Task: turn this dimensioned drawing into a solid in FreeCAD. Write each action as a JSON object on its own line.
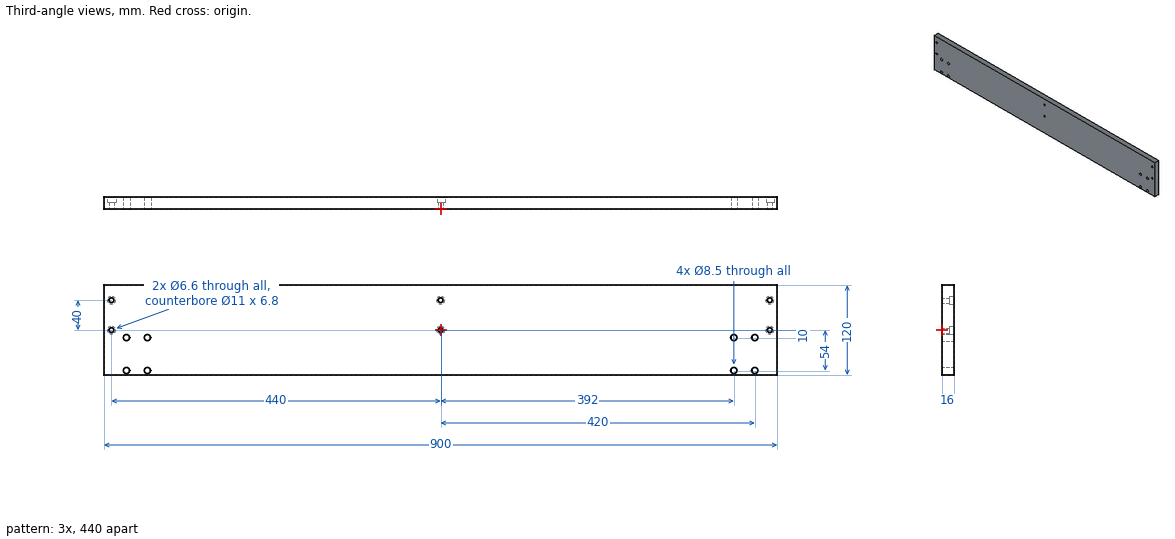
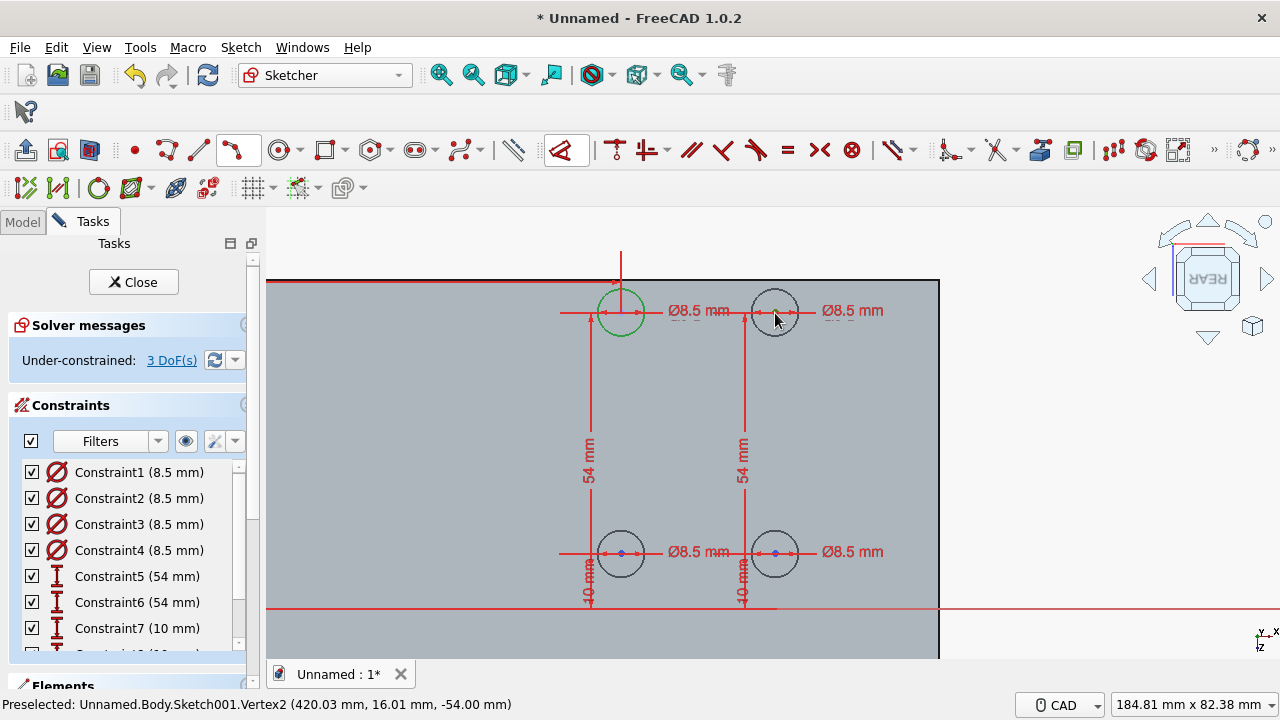
{"action": "key", "text": "l"}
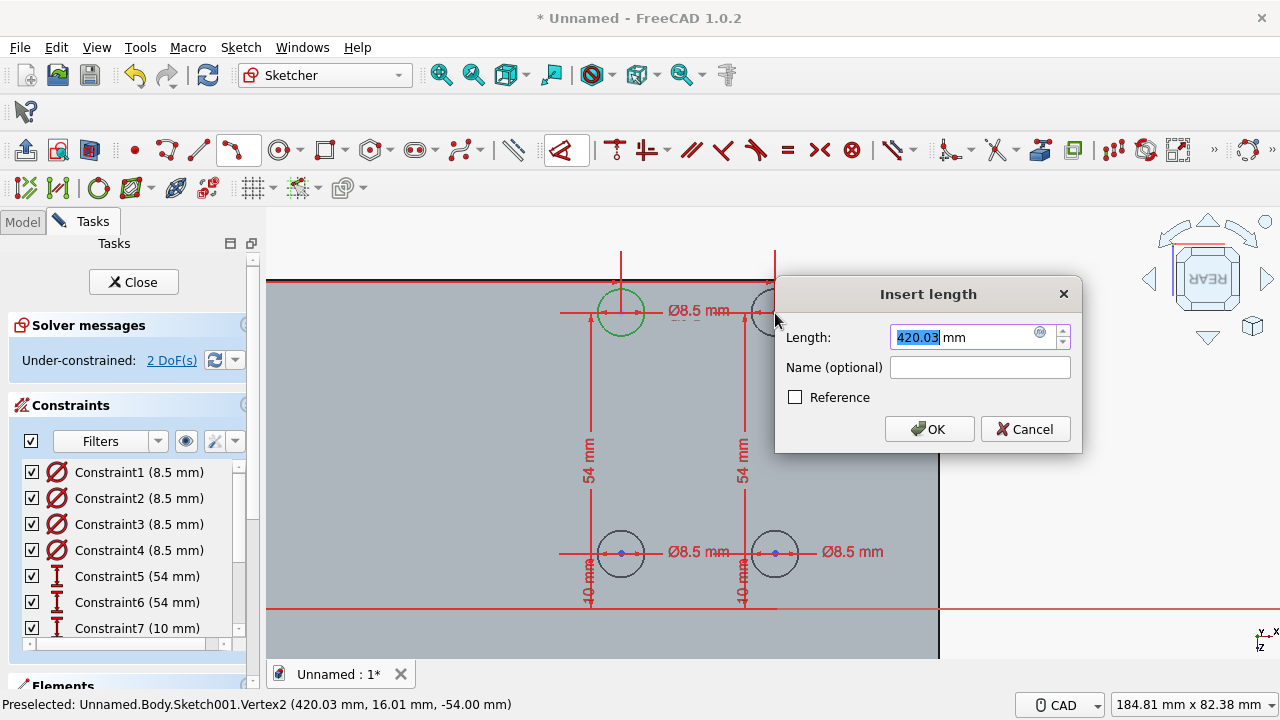
{"action": "type", "text": "420"}
{"action": "key", "text": "Return"}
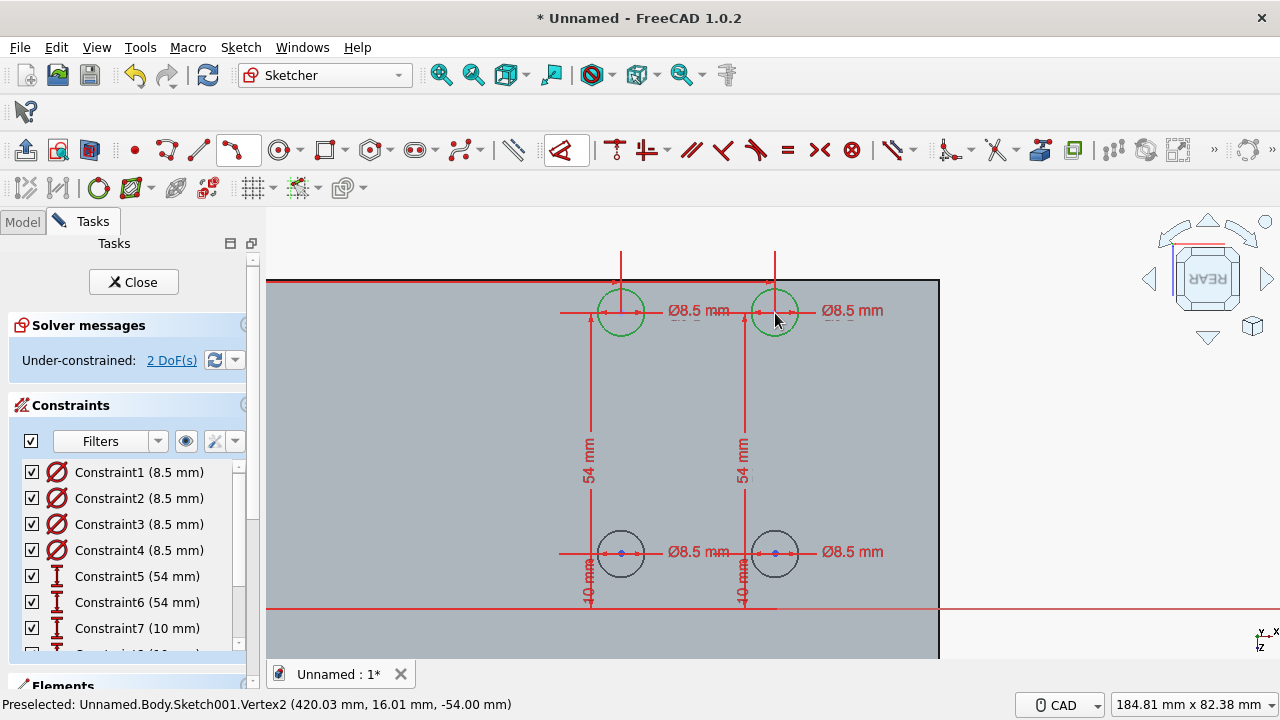
{"action": "left_click", "coordinate": [621, 554]}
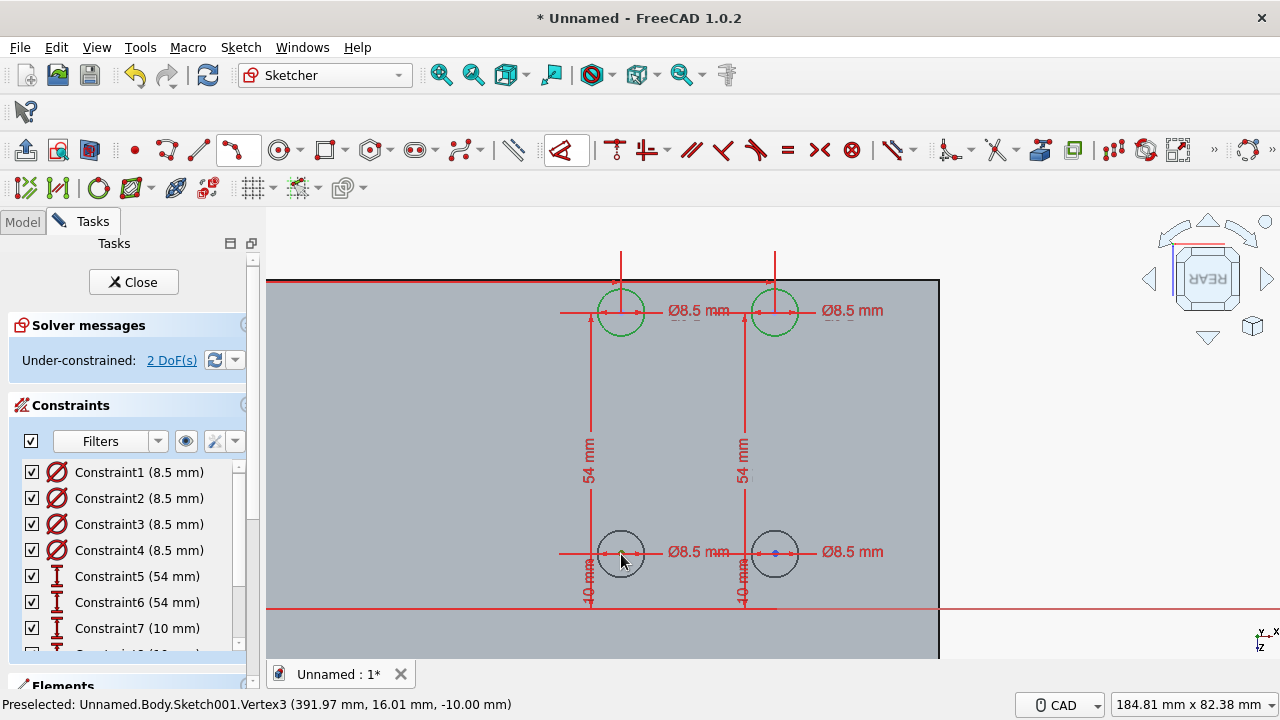
{"action": "key", "text": "l"}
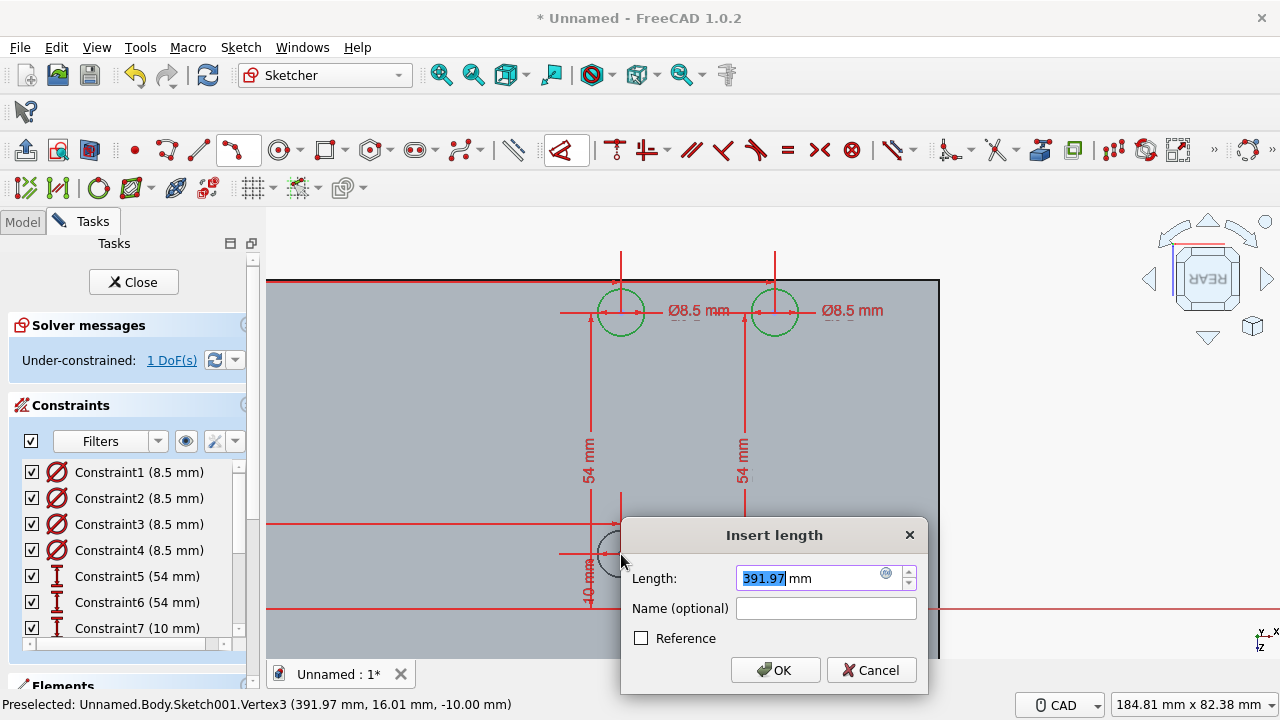
{"action": "type", "text": "392"}
{"action": "key", "text": "Return"}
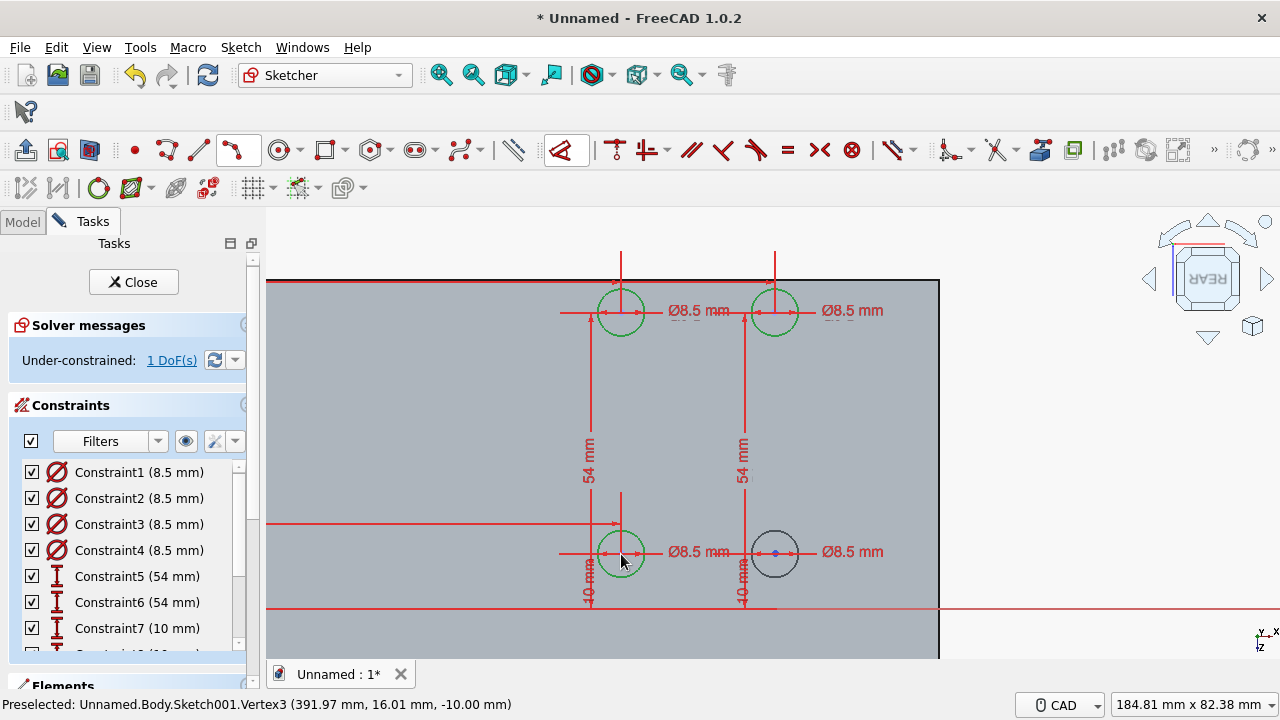
{"action": "left_click", "coordinate": [775, 554]}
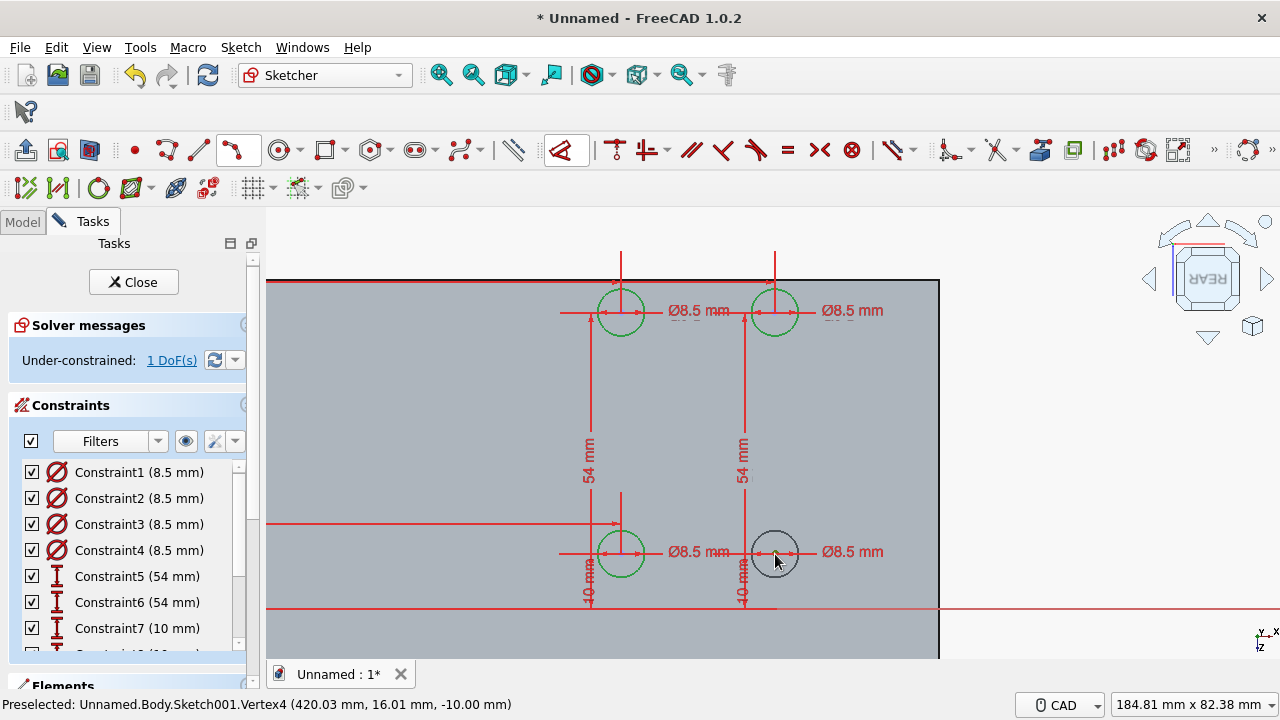
{"action": "key", "text": "l"}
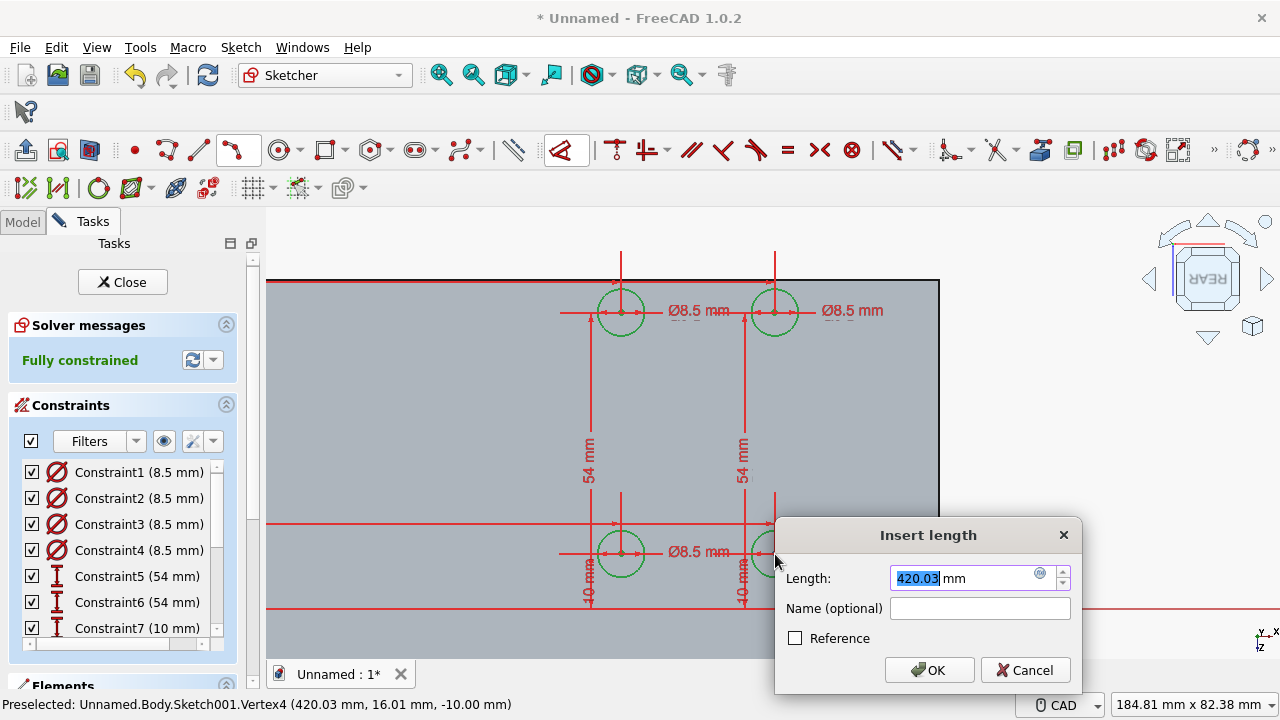
{"action": "type", "text": "420"}
{"action": "key", "text": "Return"}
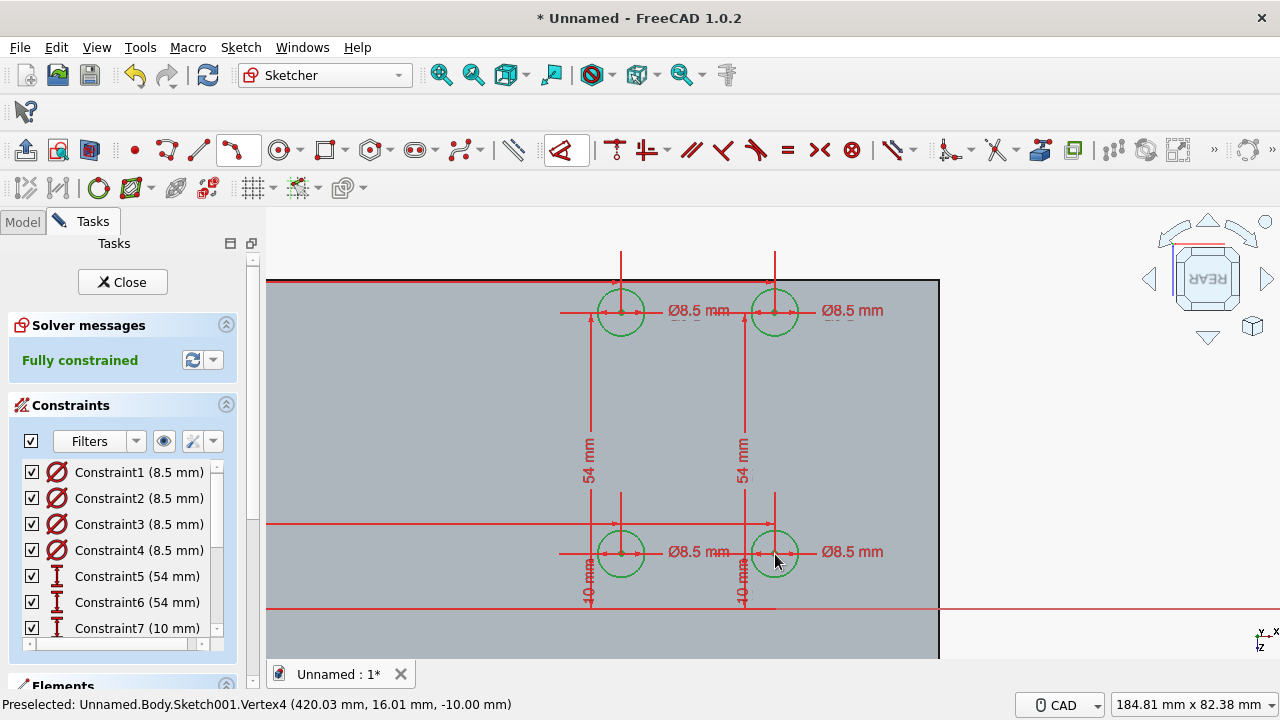
{"action": "left_click", "coordinate": [123, 282]}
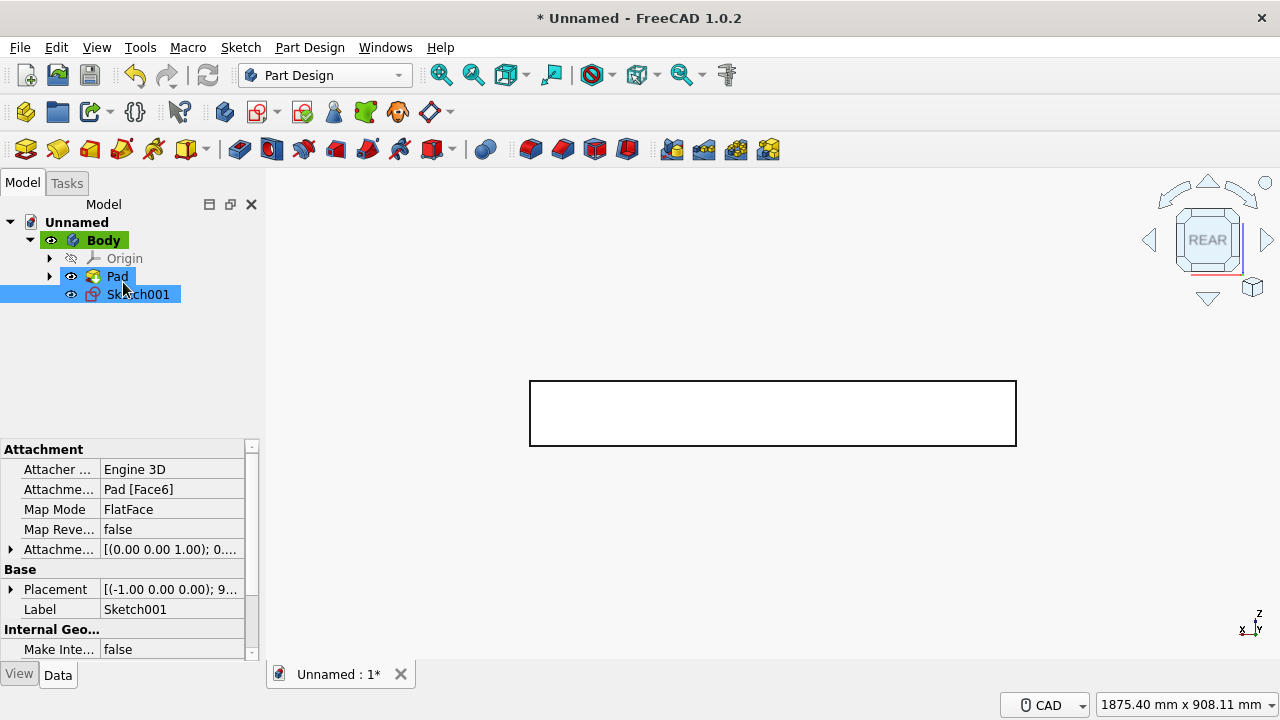
{"action": "left_click", "coordinate": [272, 150]}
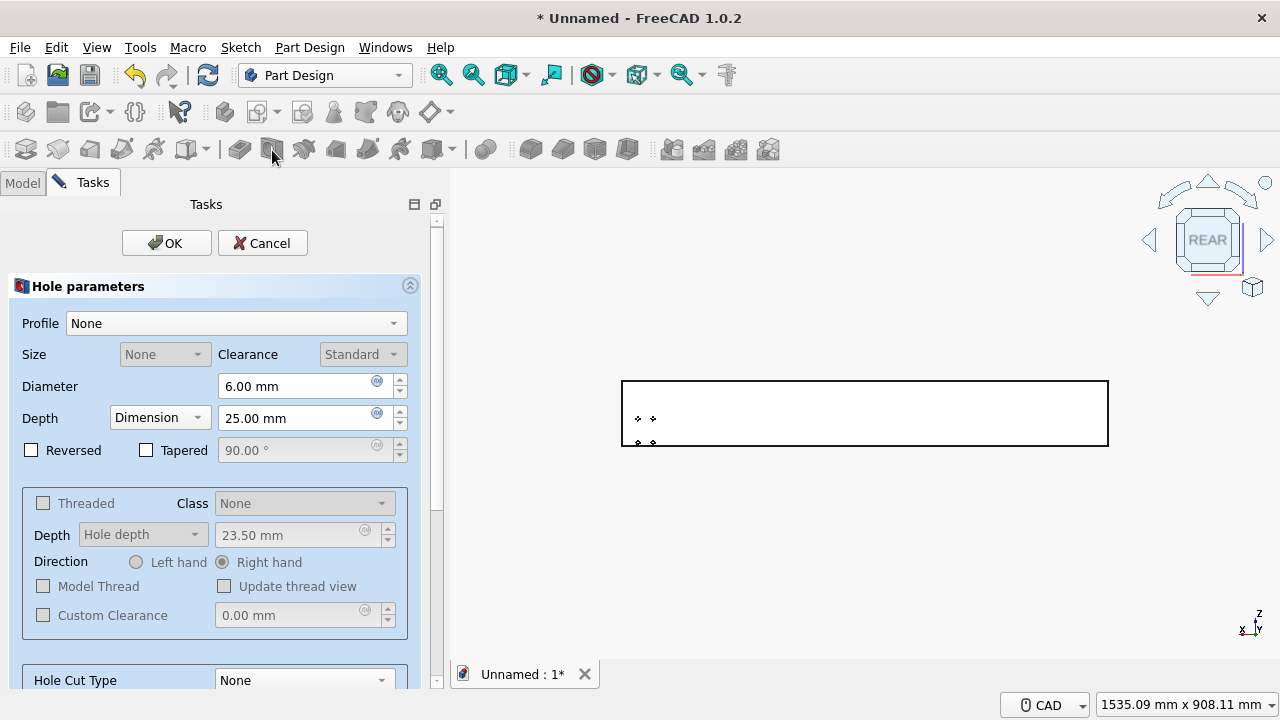
{"action": "triple_click", "coordinate": [305, 386]}